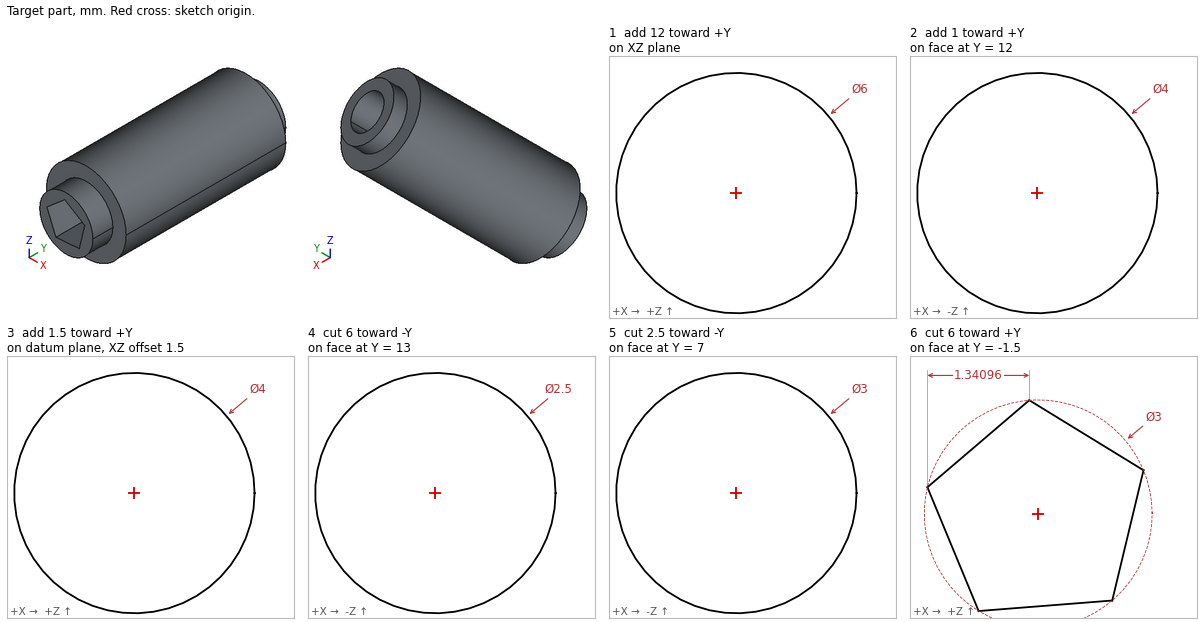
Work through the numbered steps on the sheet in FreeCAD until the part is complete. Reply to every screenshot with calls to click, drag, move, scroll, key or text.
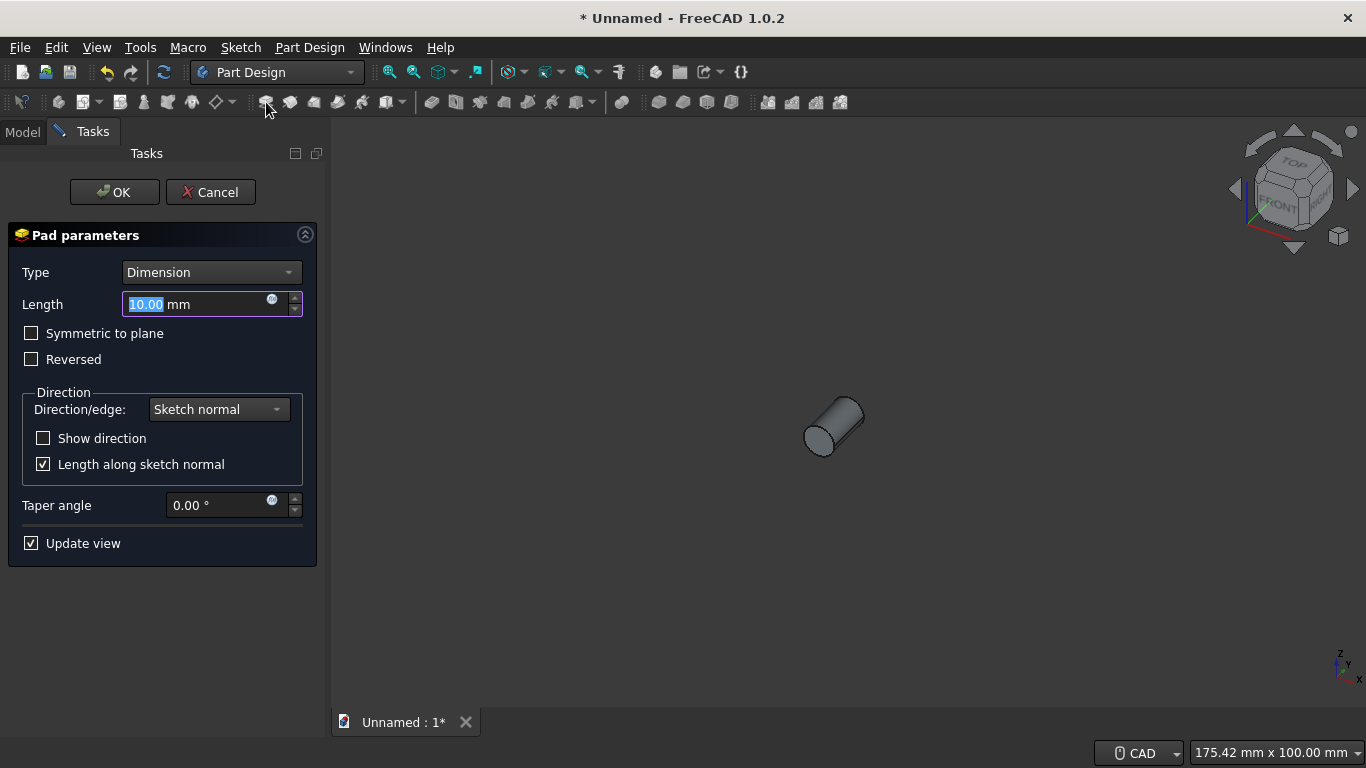
text(12)
key(Tab)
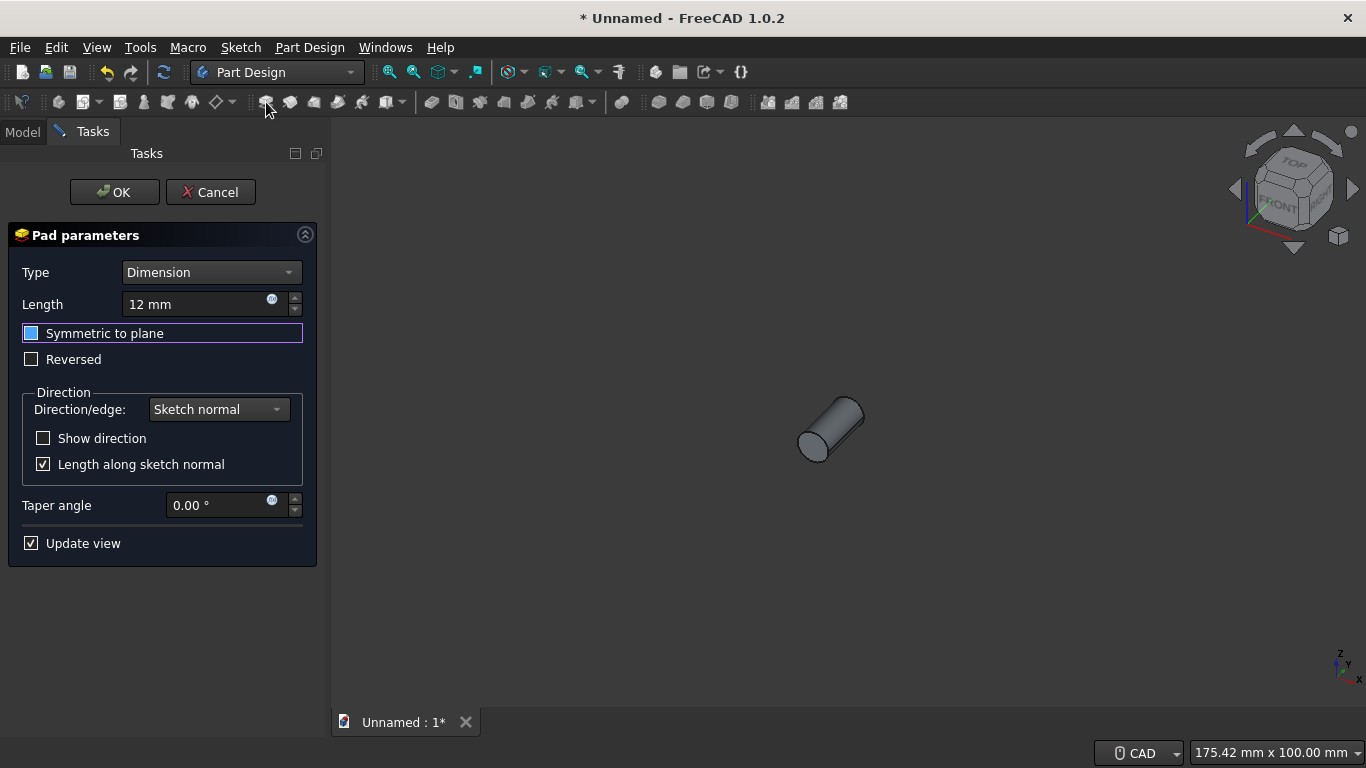
click(30, 359)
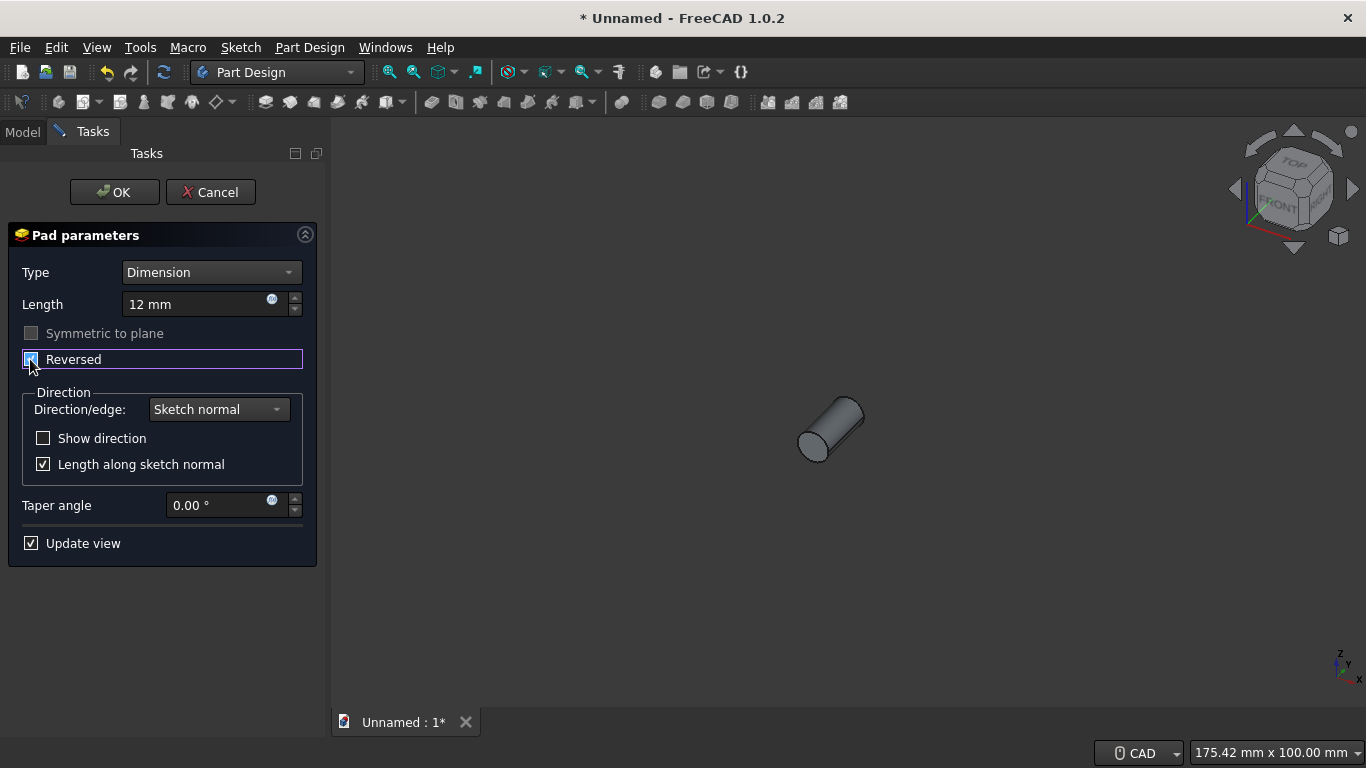
click(115, 192)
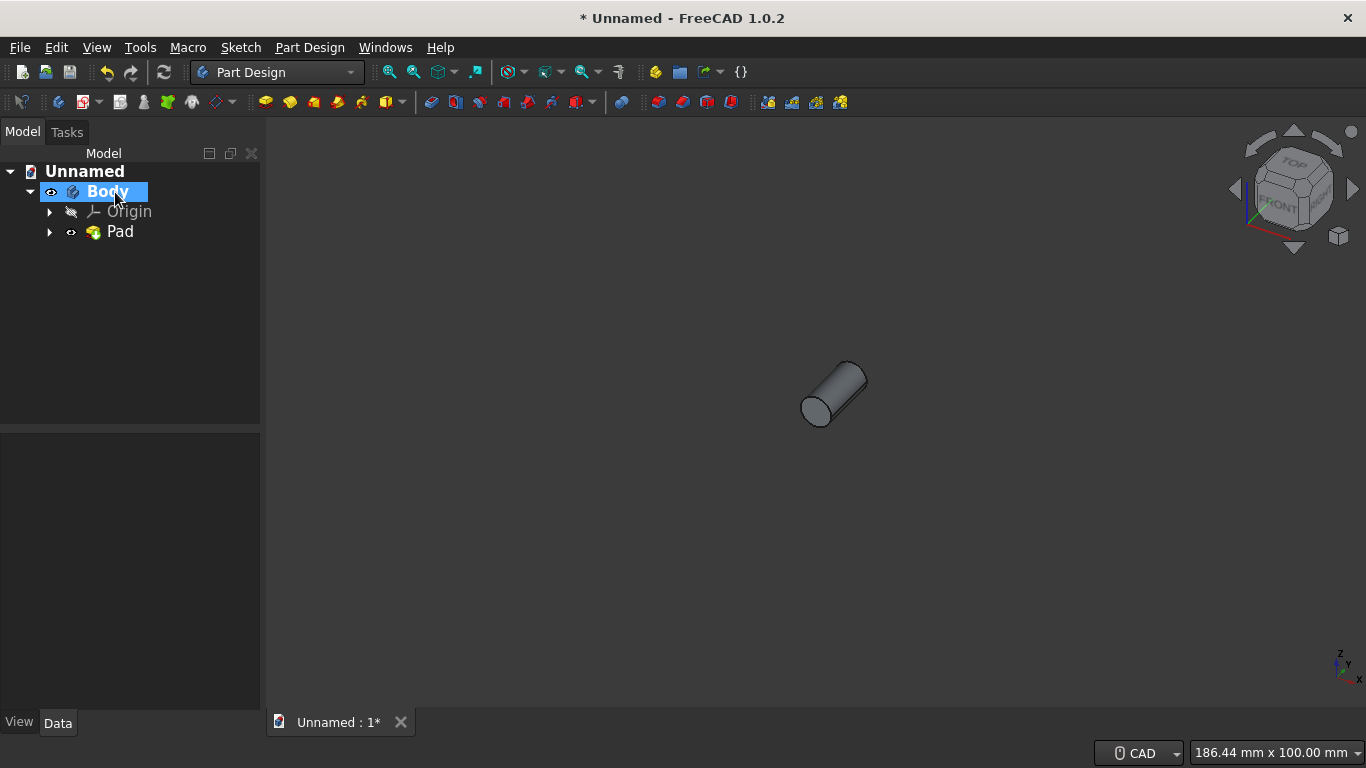
click(390, 72)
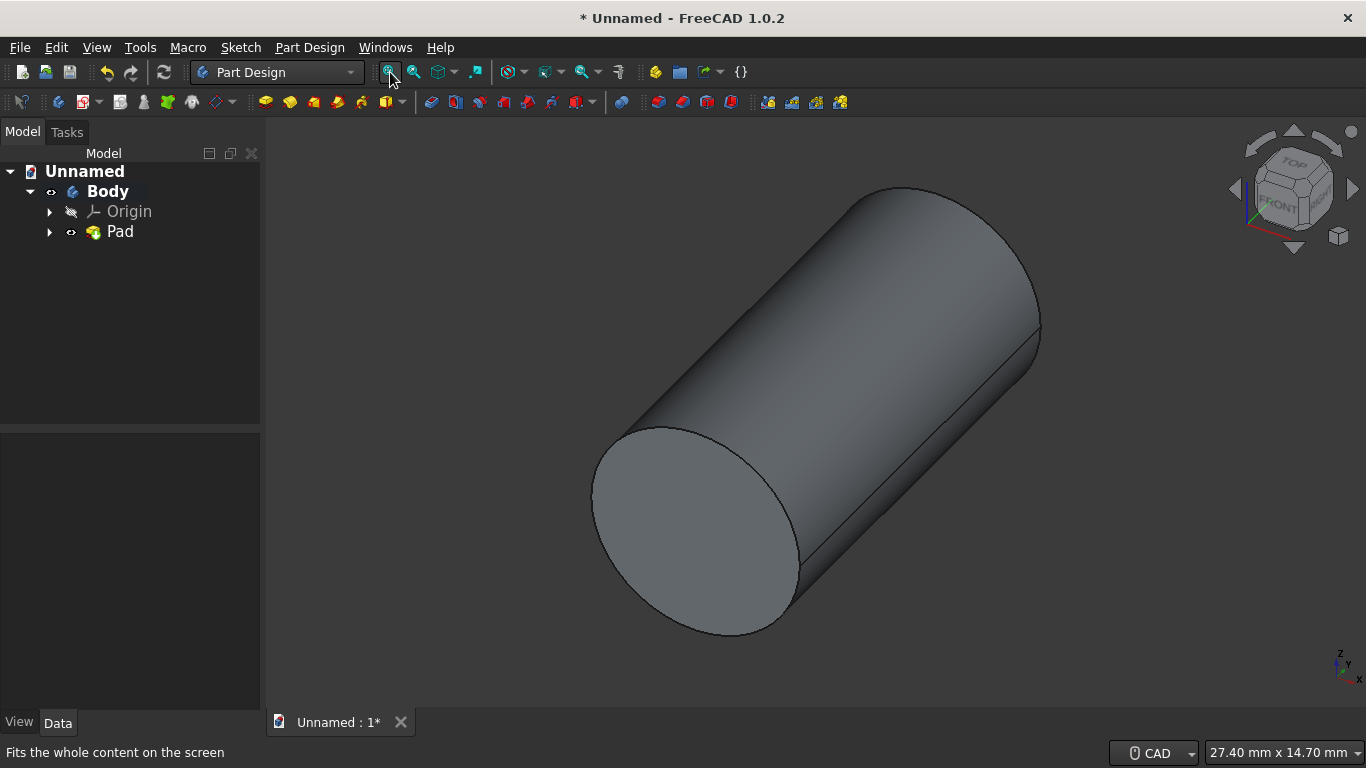
key(4)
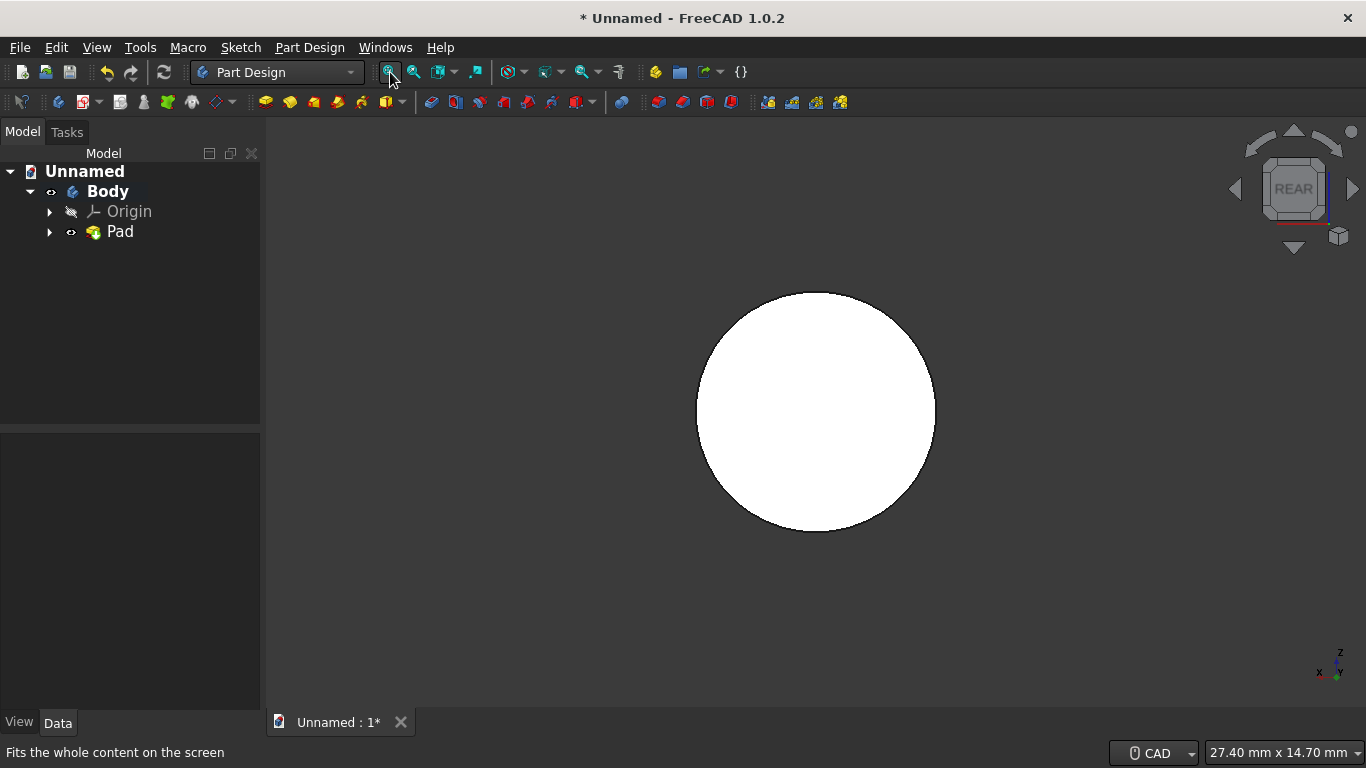
click(390, 72)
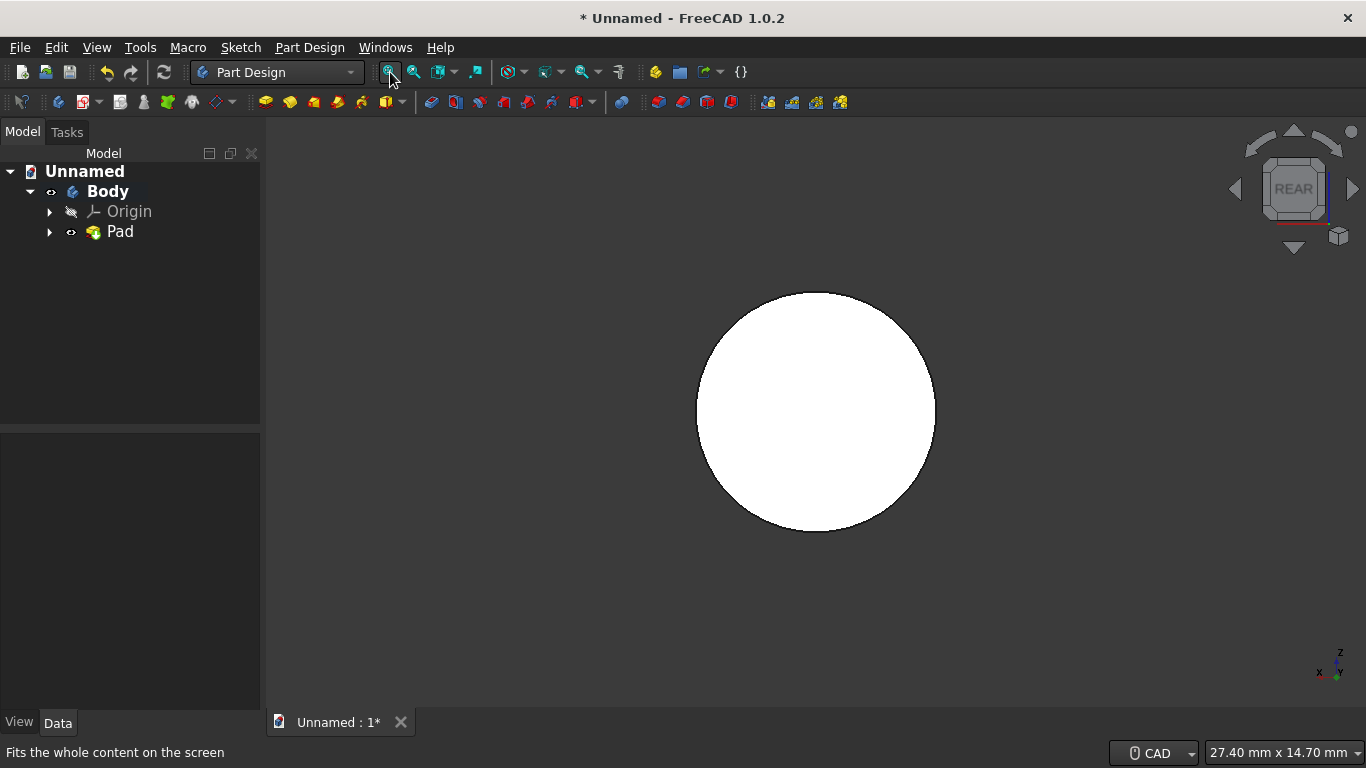
click(816, 411)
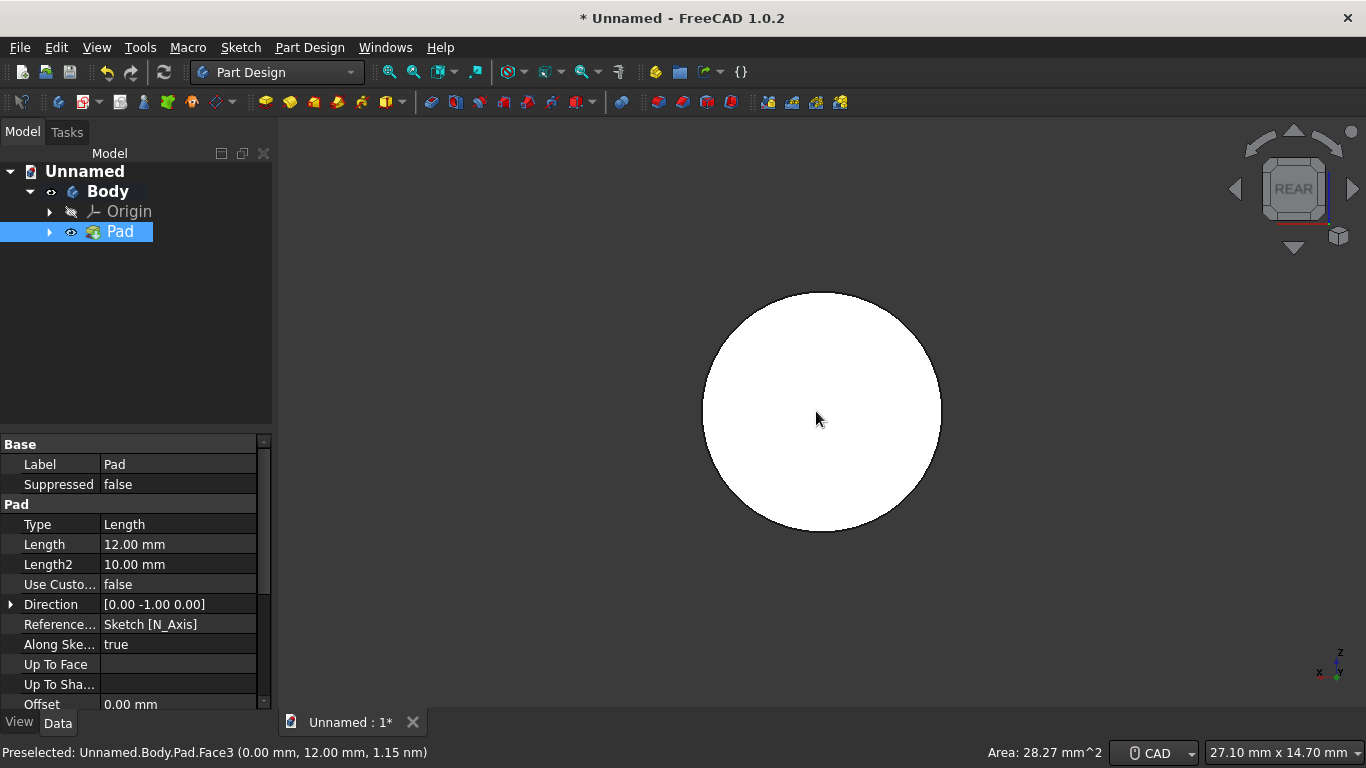
click(84, 102)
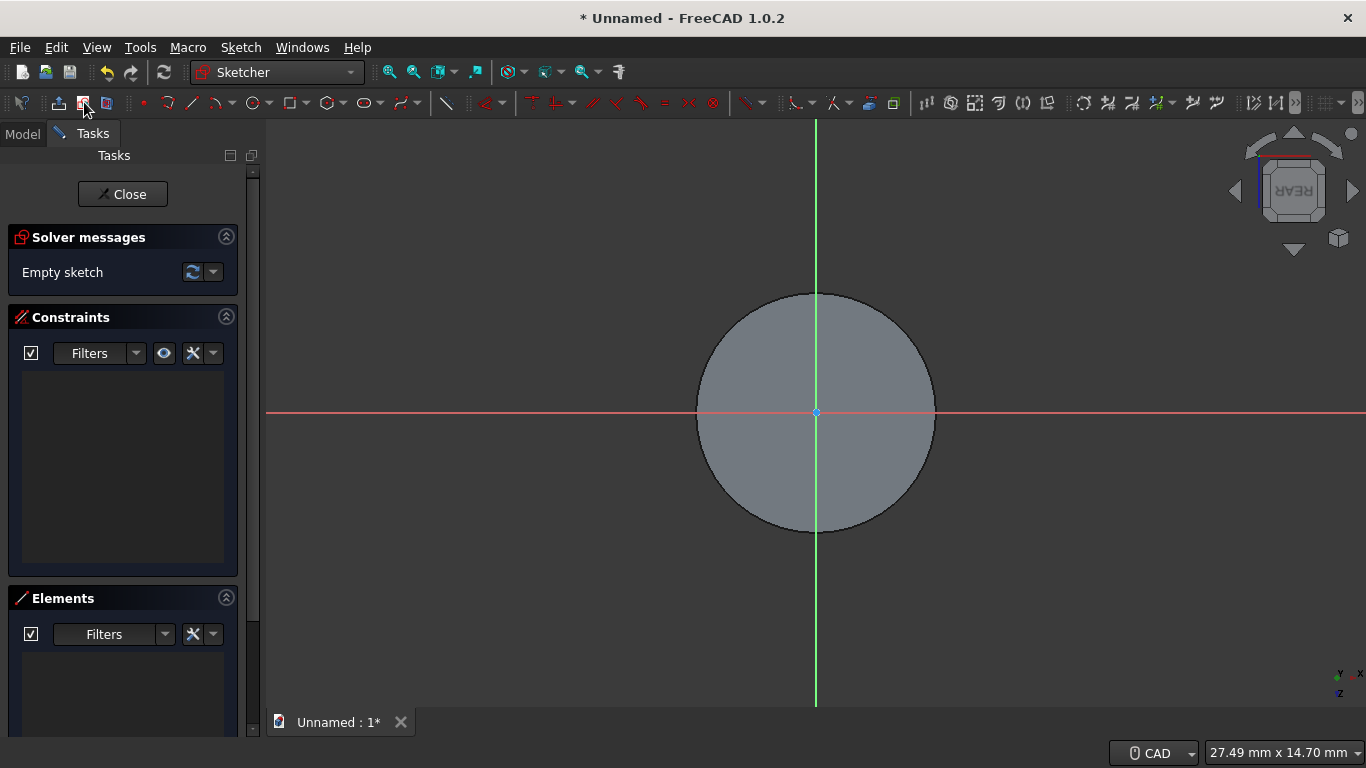
scroll(872, 413, up, 4)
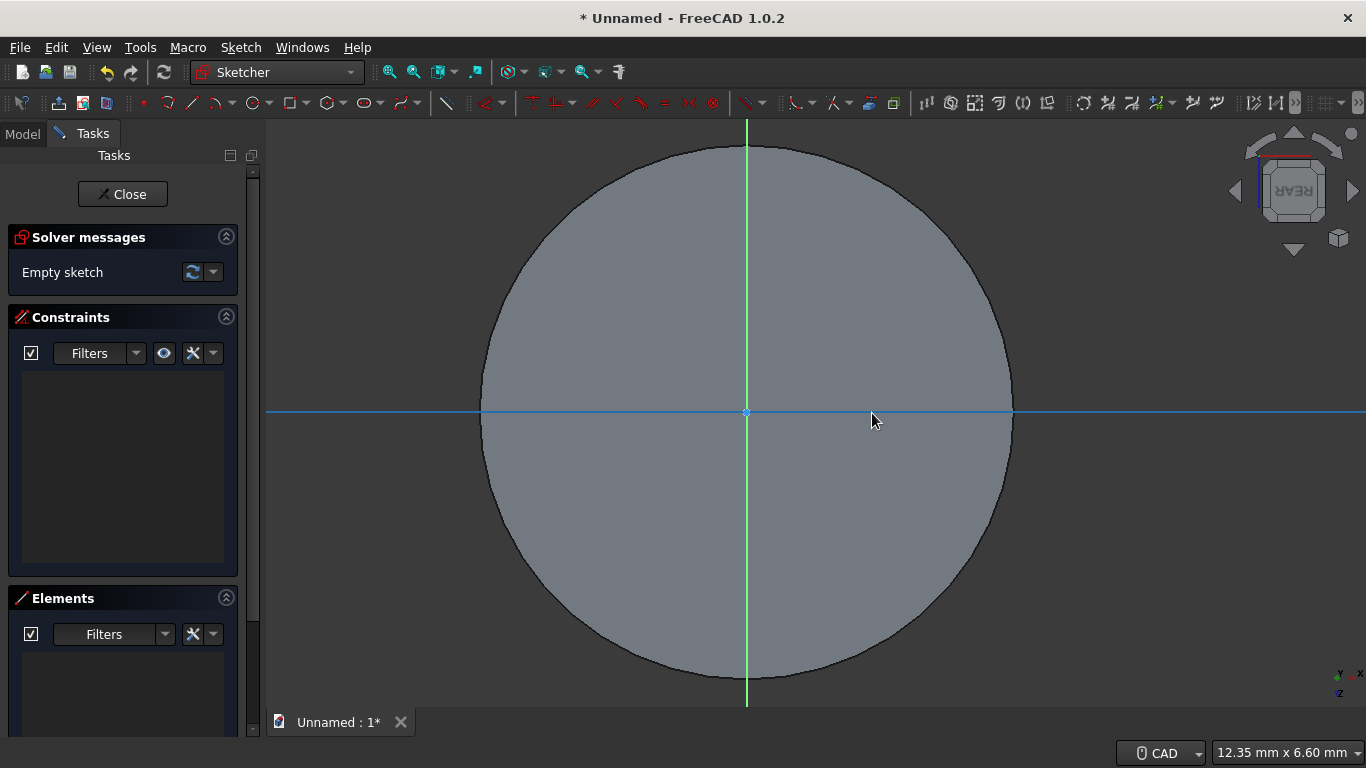
click(254, 104)